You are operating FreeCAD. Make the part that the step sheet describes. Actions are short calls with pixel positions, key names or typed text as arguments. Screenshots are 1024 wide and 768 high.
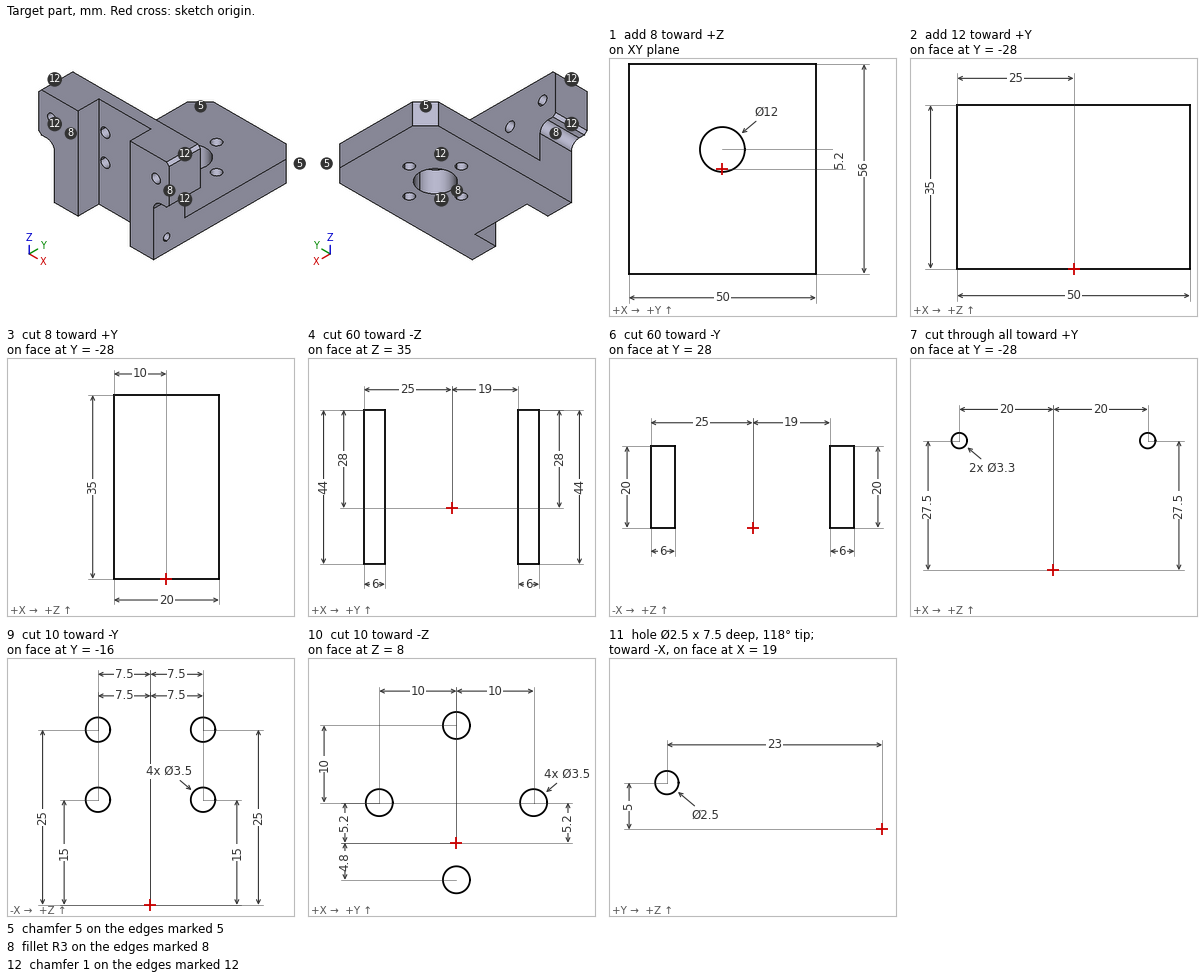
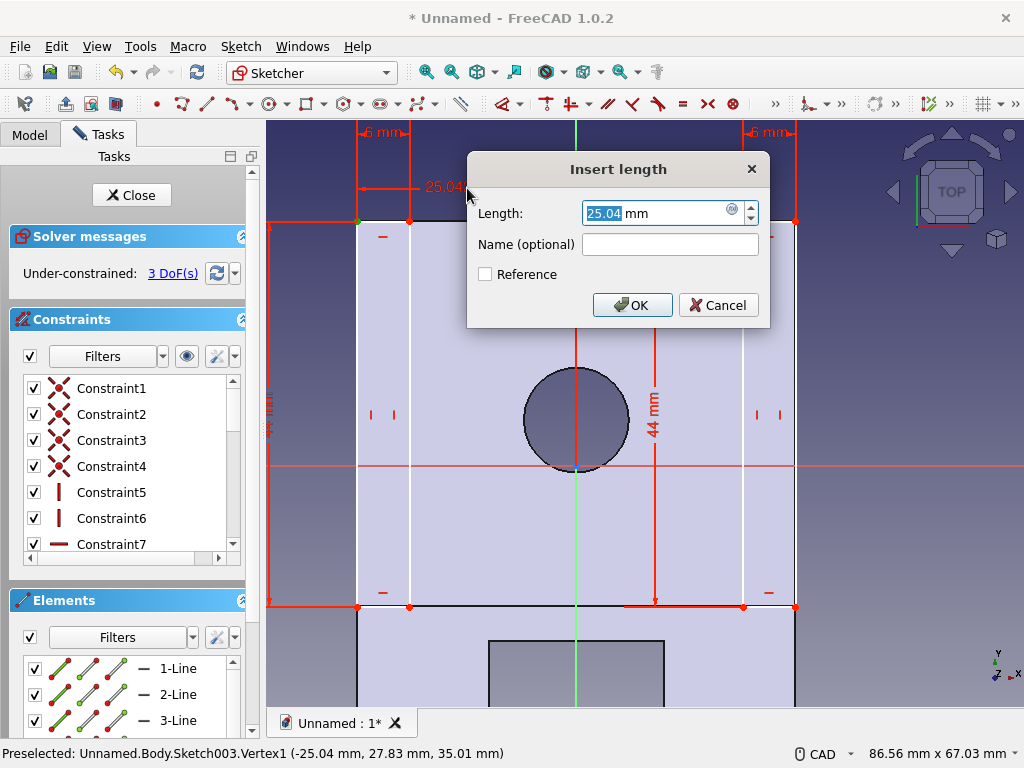
text(25)
key(Return)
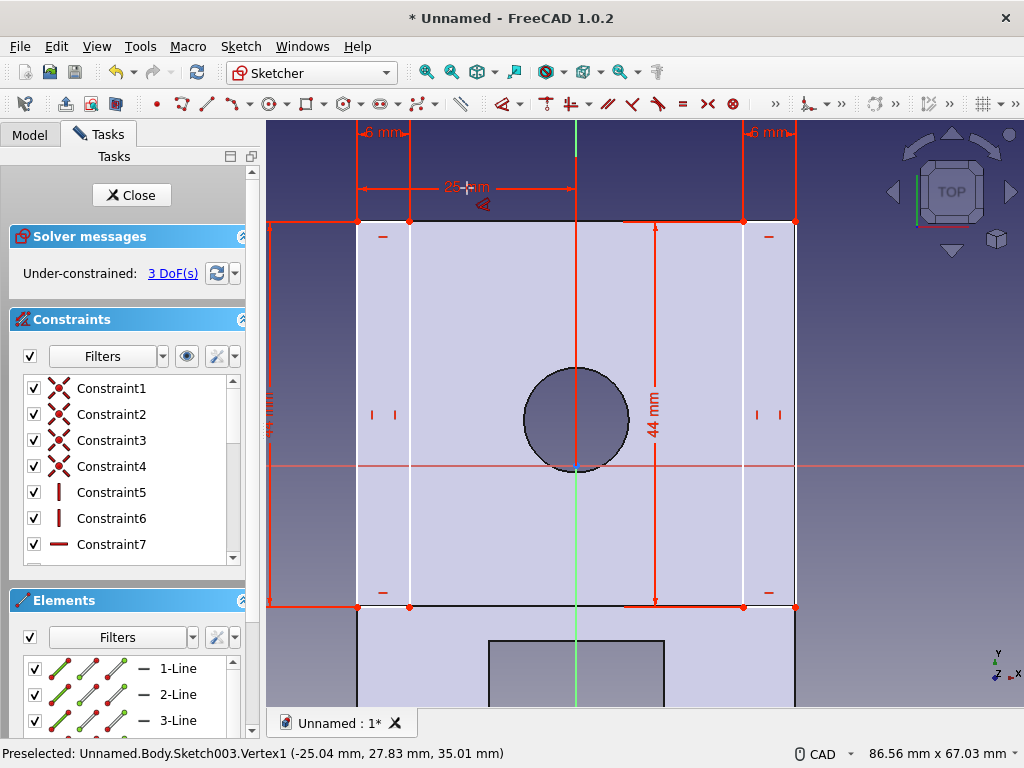
click(357, 222)
click(323, 344)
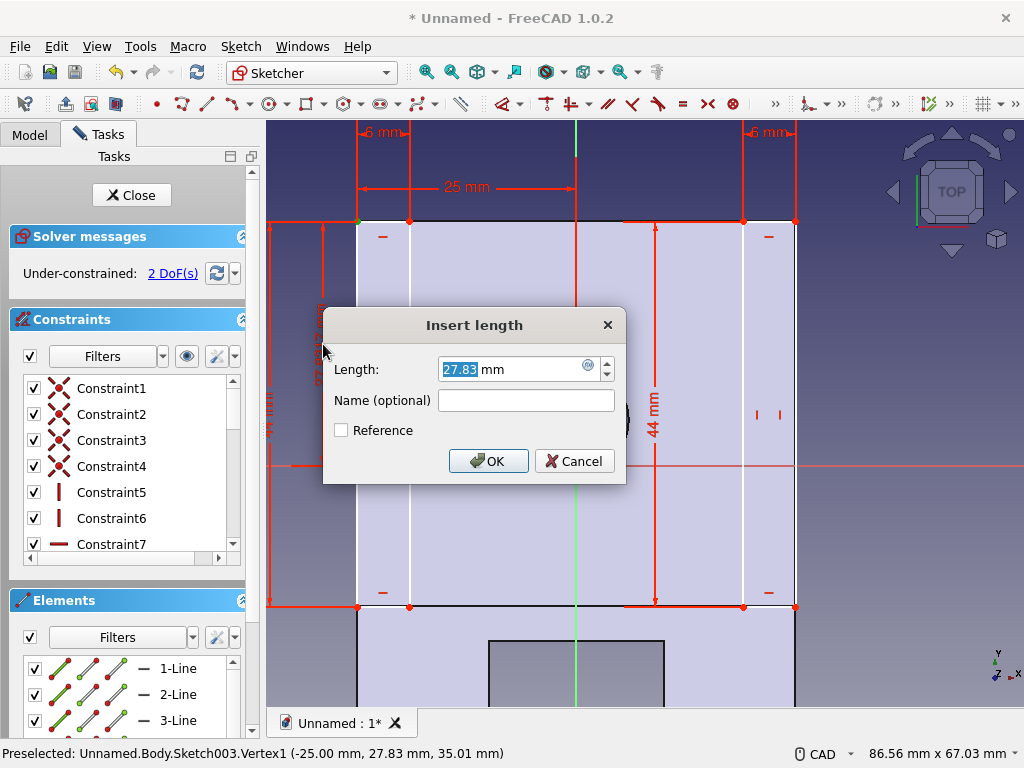
text(28)
key(Return)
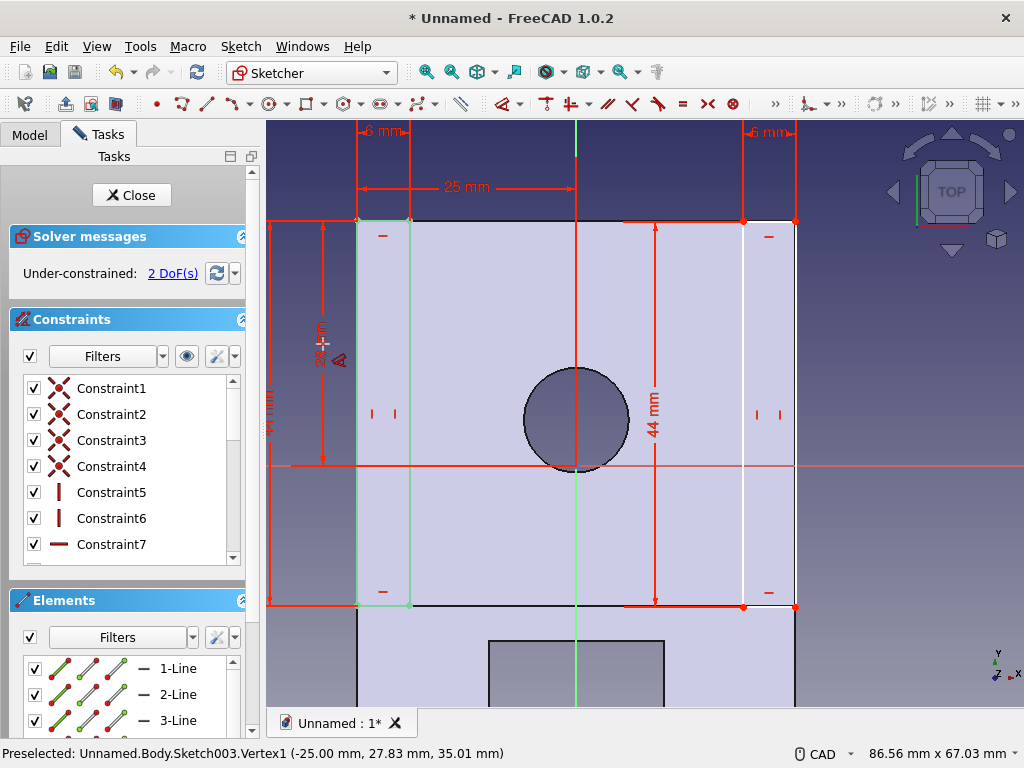
click(743, 222)
click(660, 188)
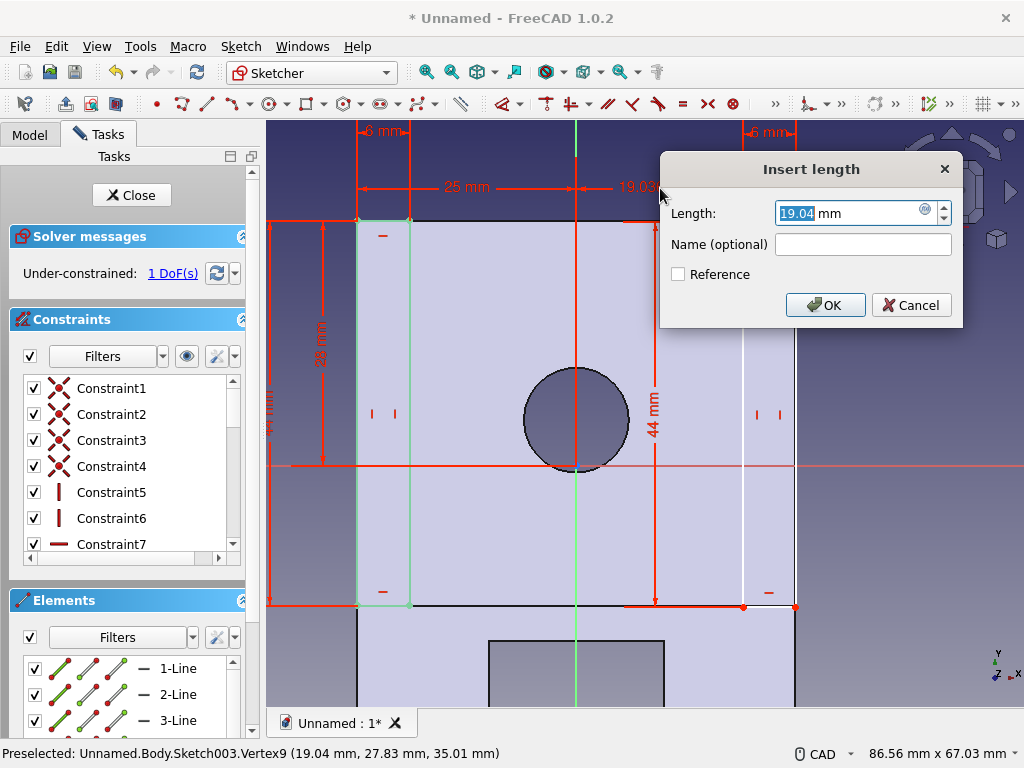
text(19)
key(Return)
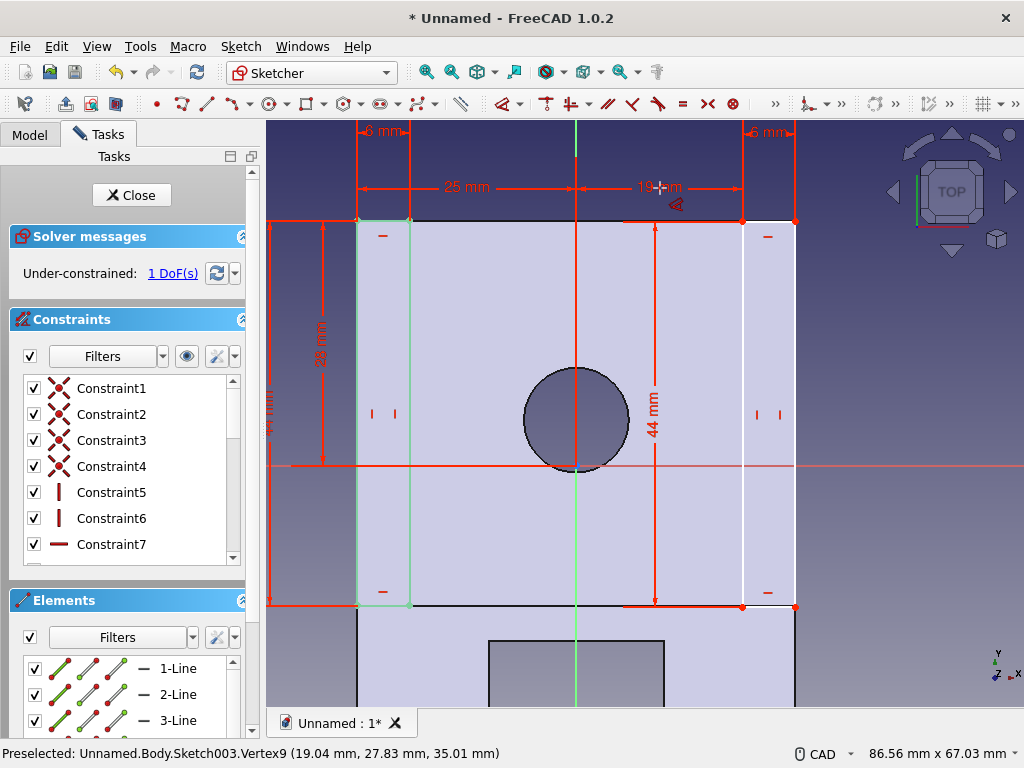
click(743, 222)
click(777, 344)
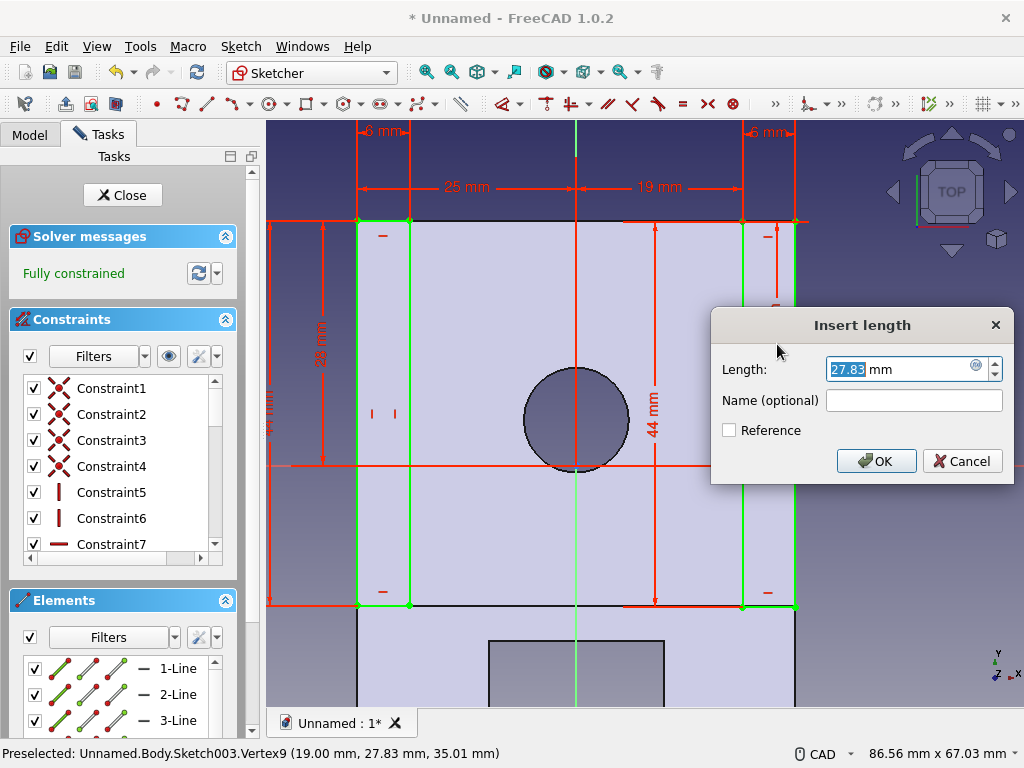
text(28)
key(Return)
key(Escape)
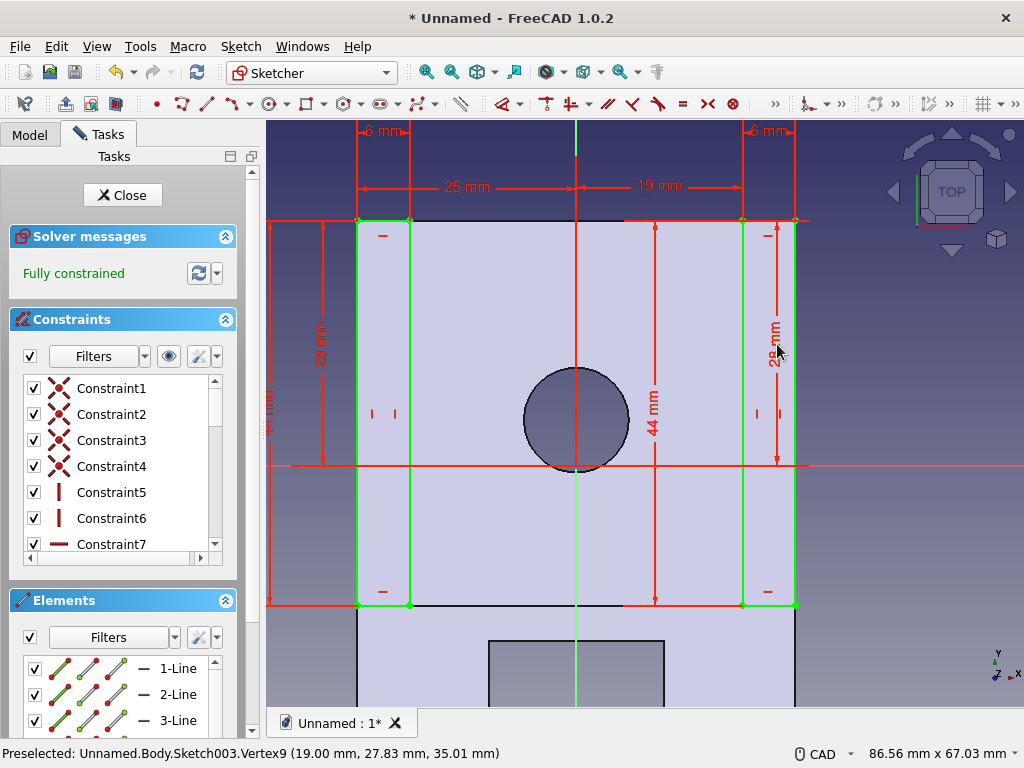
click(123, 195)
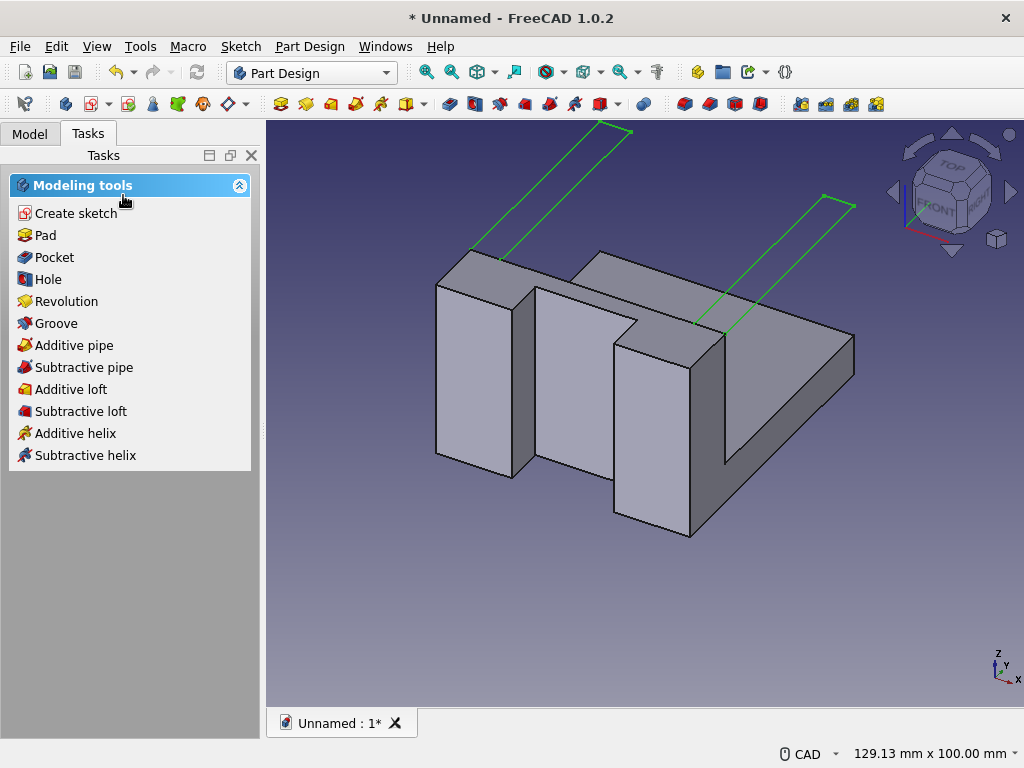
click(450, 104)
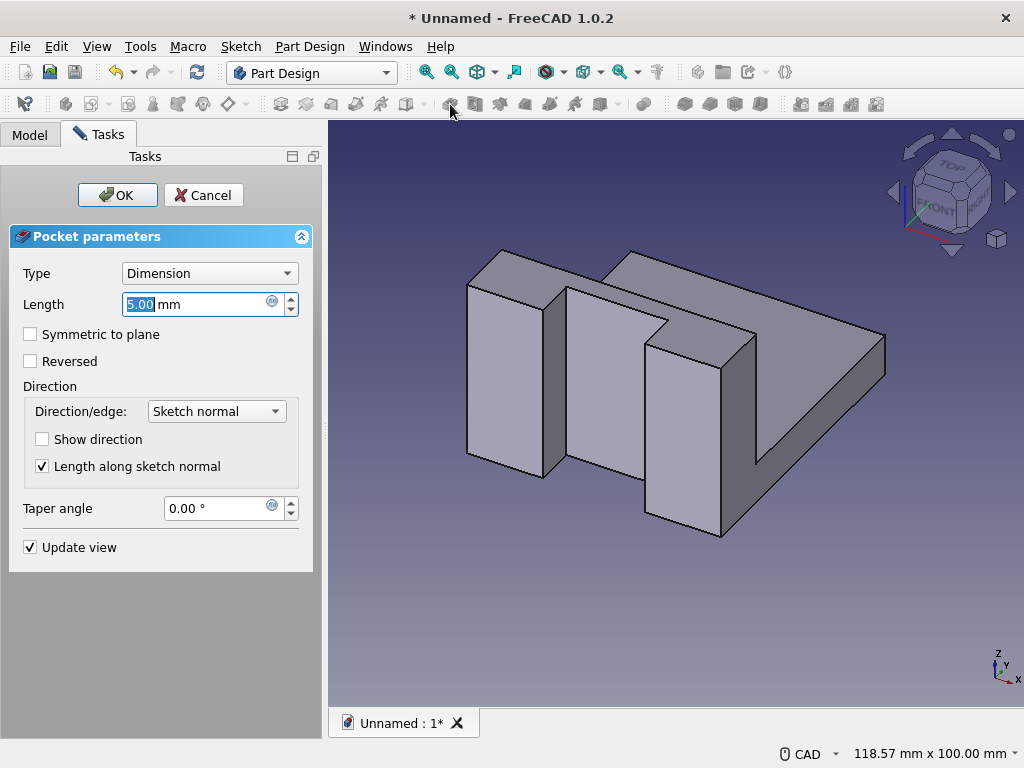
text(60)
key(Tab)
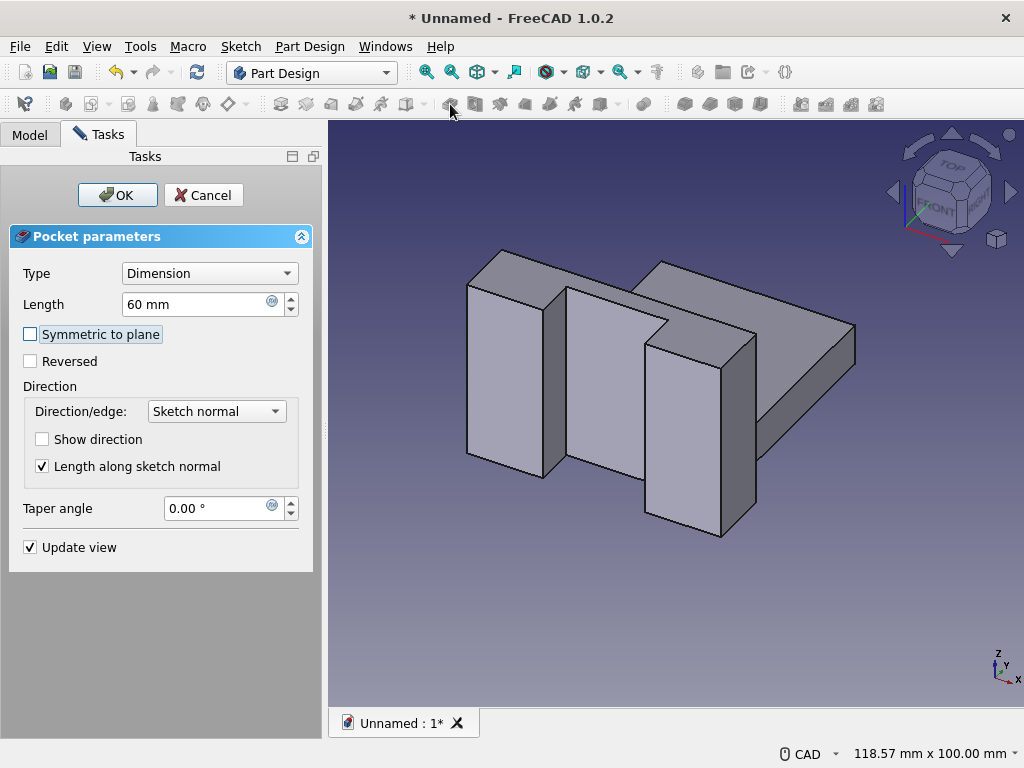
click(118, 195)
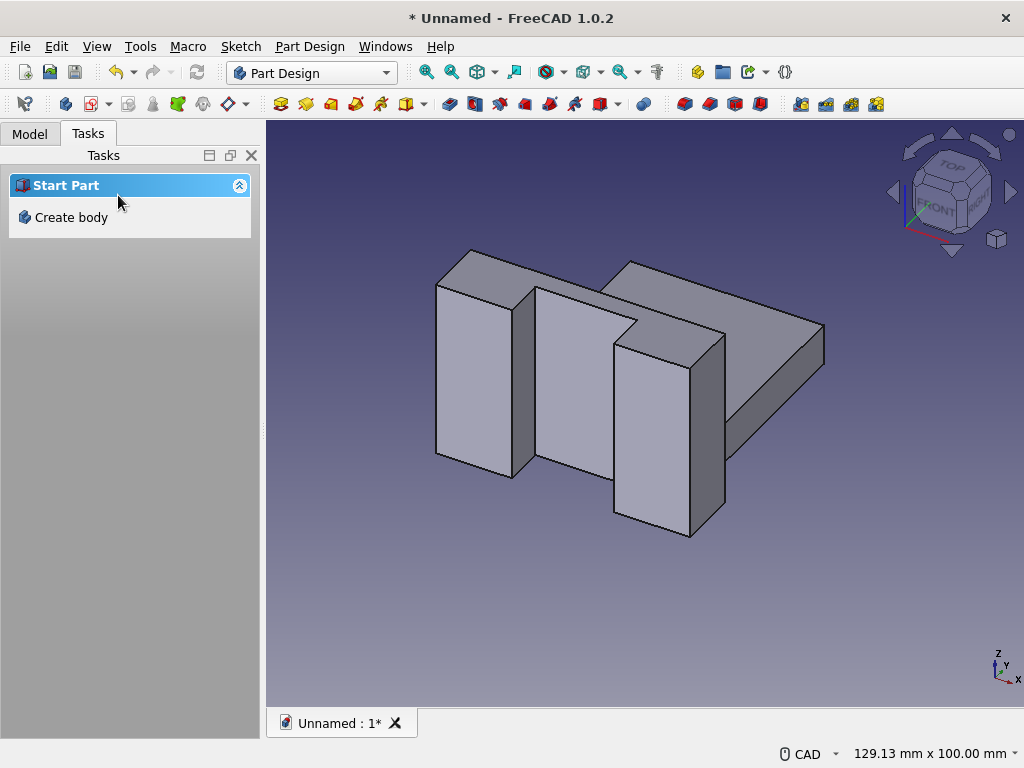
key(0)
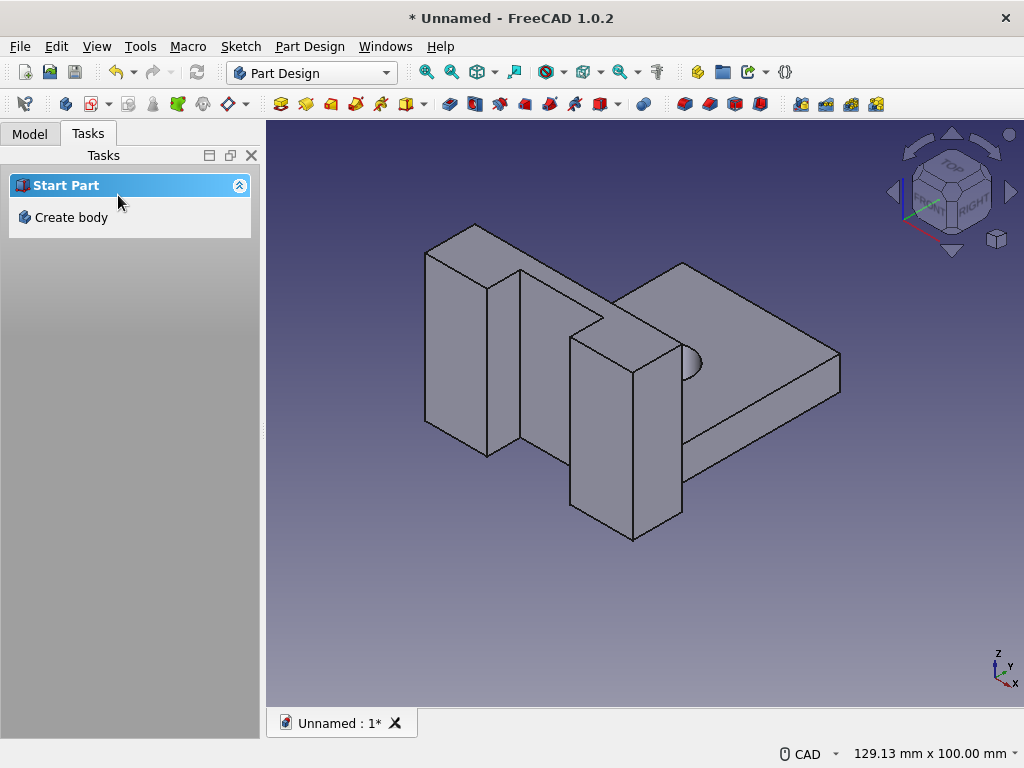
click(427, 72)